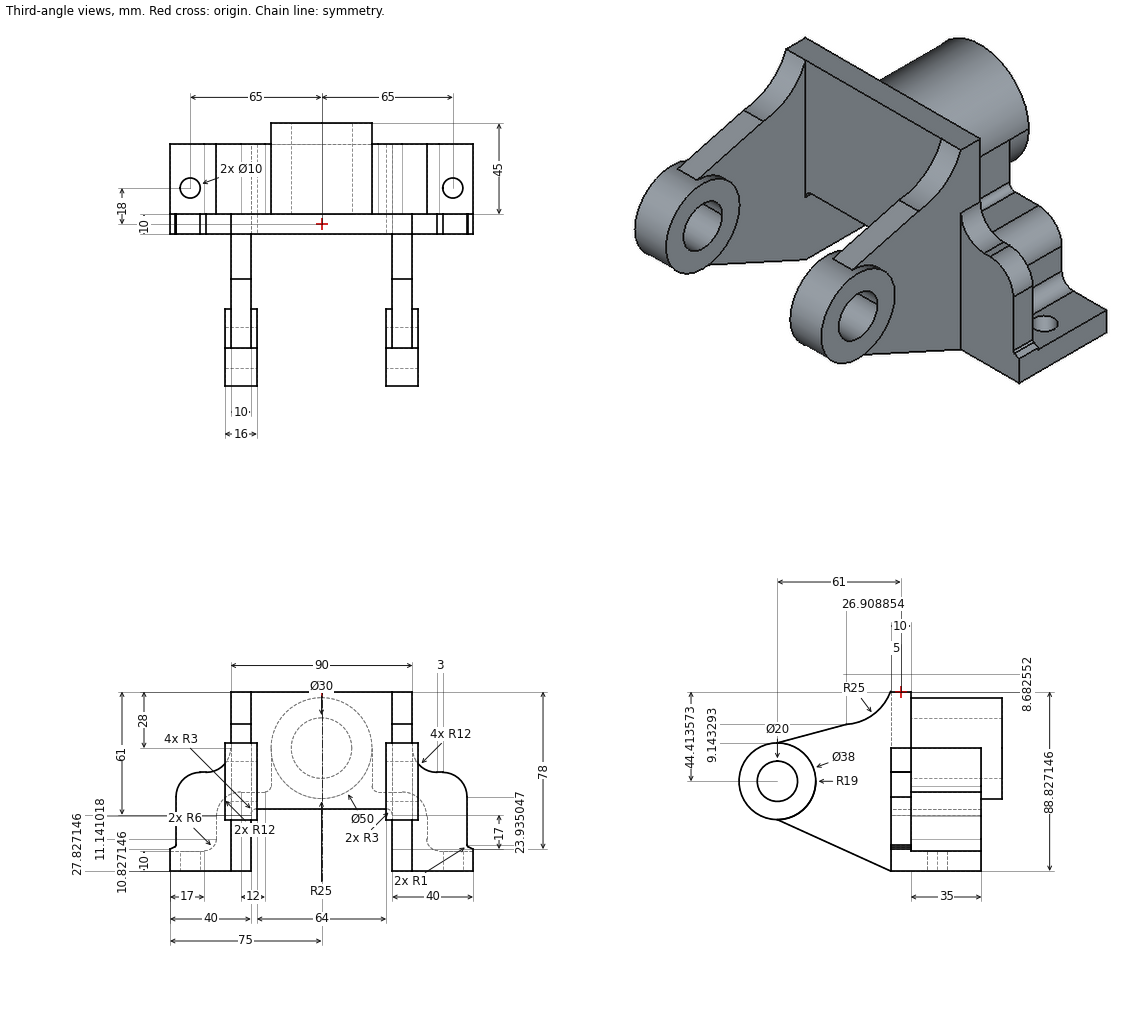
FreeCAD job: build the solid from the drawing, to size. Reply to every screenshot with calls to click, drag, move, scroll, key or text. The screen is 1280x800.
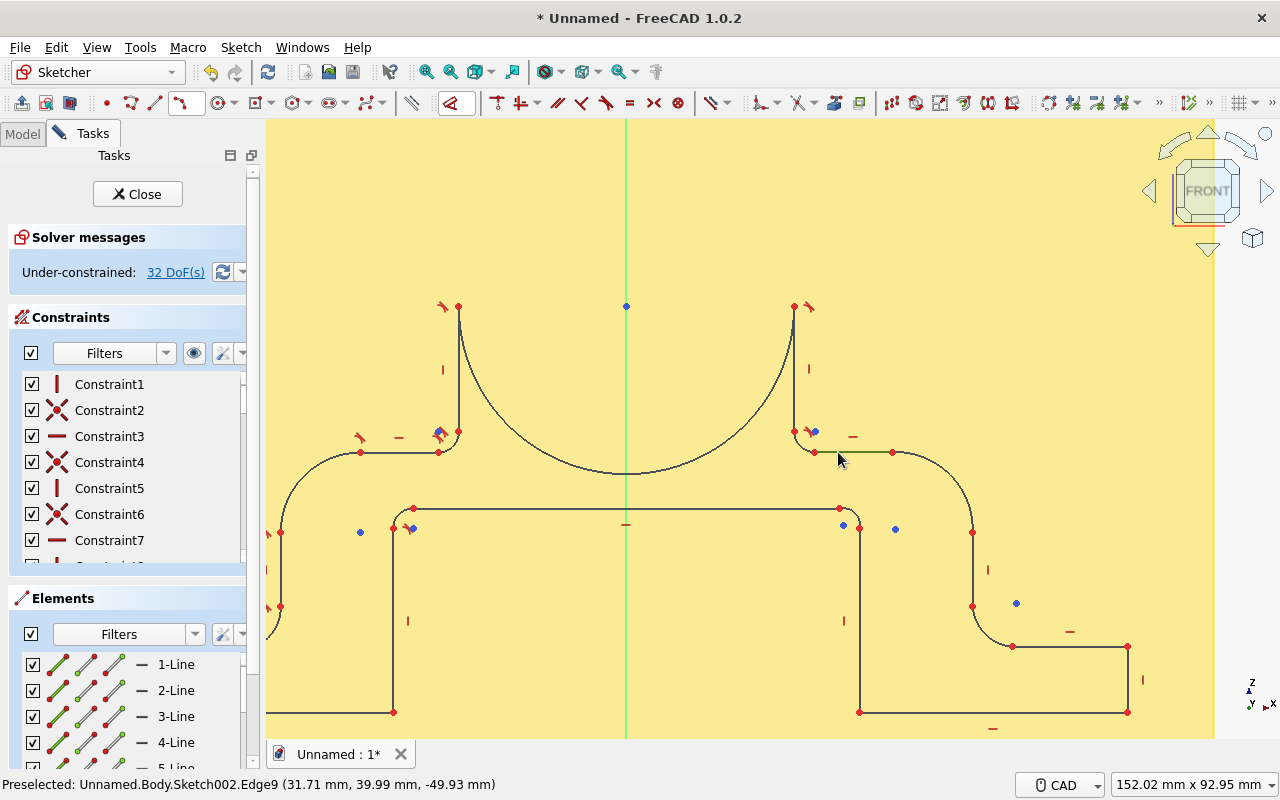
scroll(796, 440, up, 2)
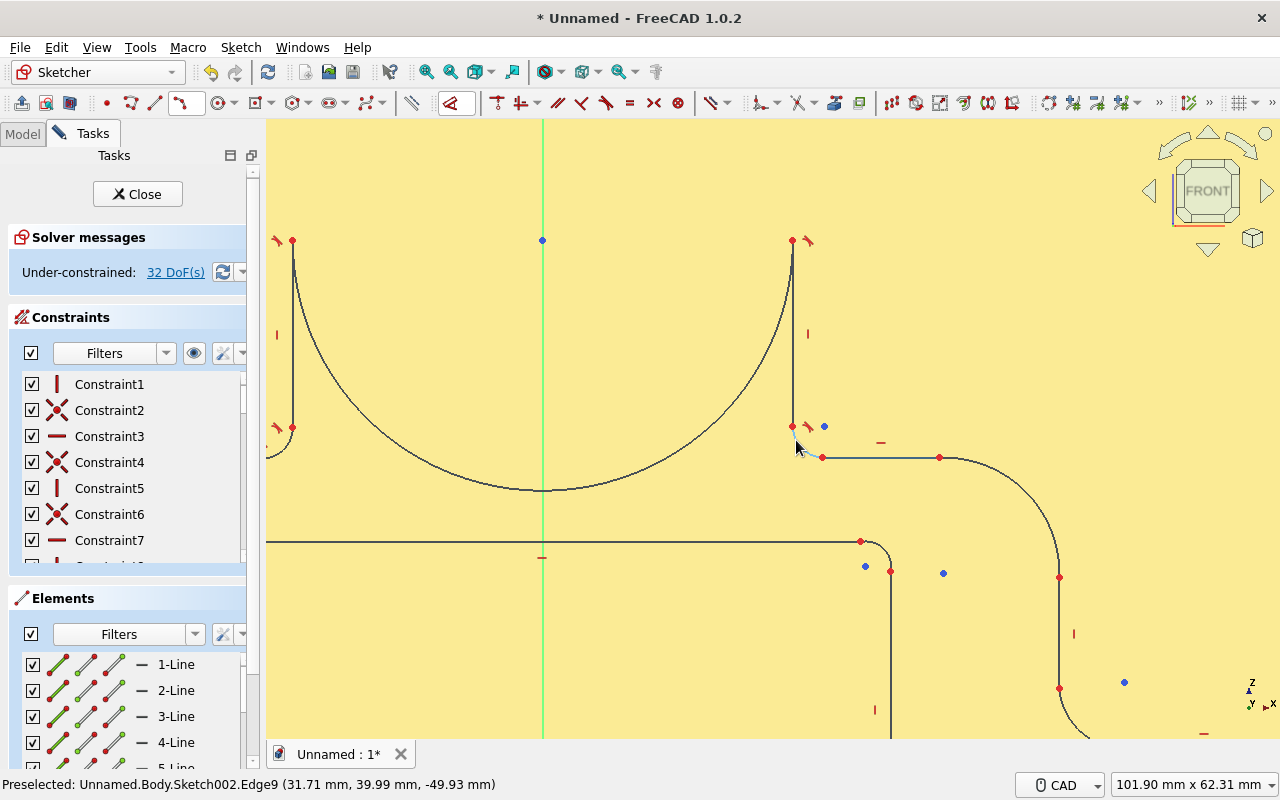
click(796, 440)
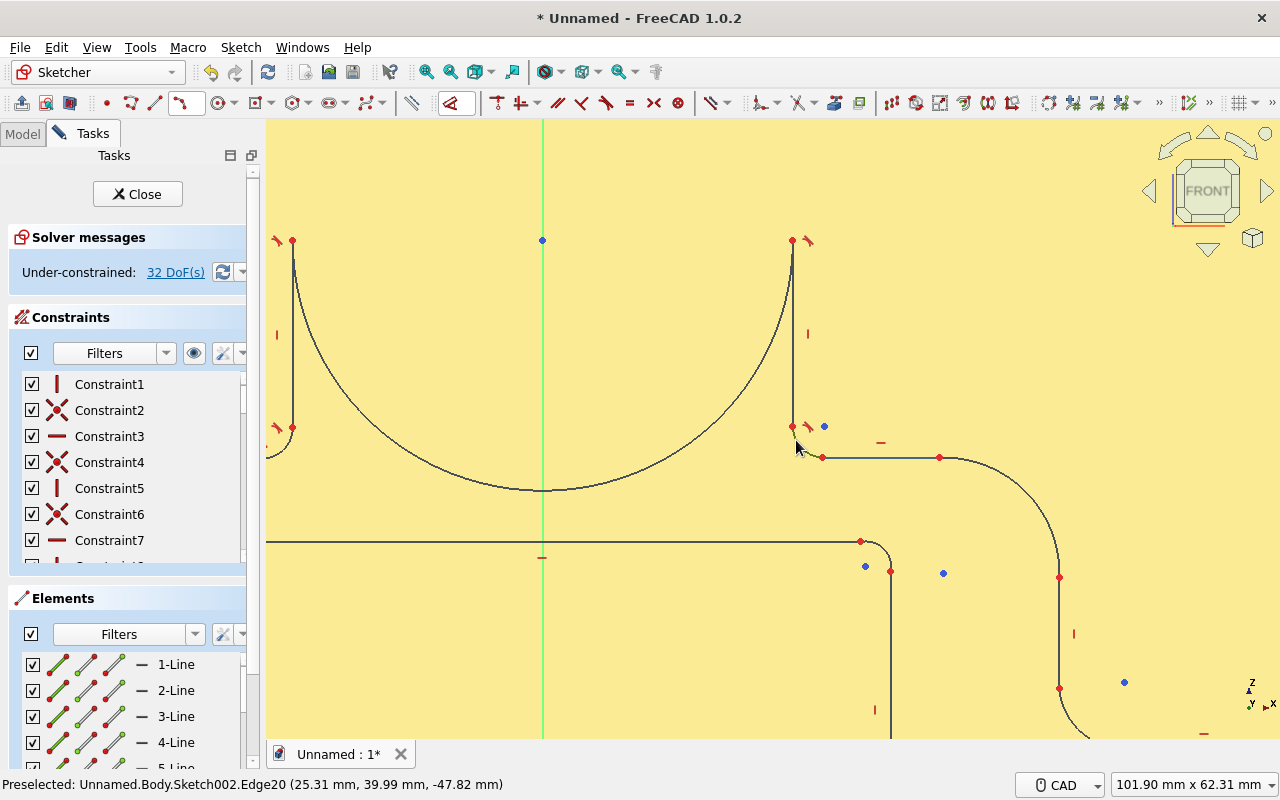
key(t)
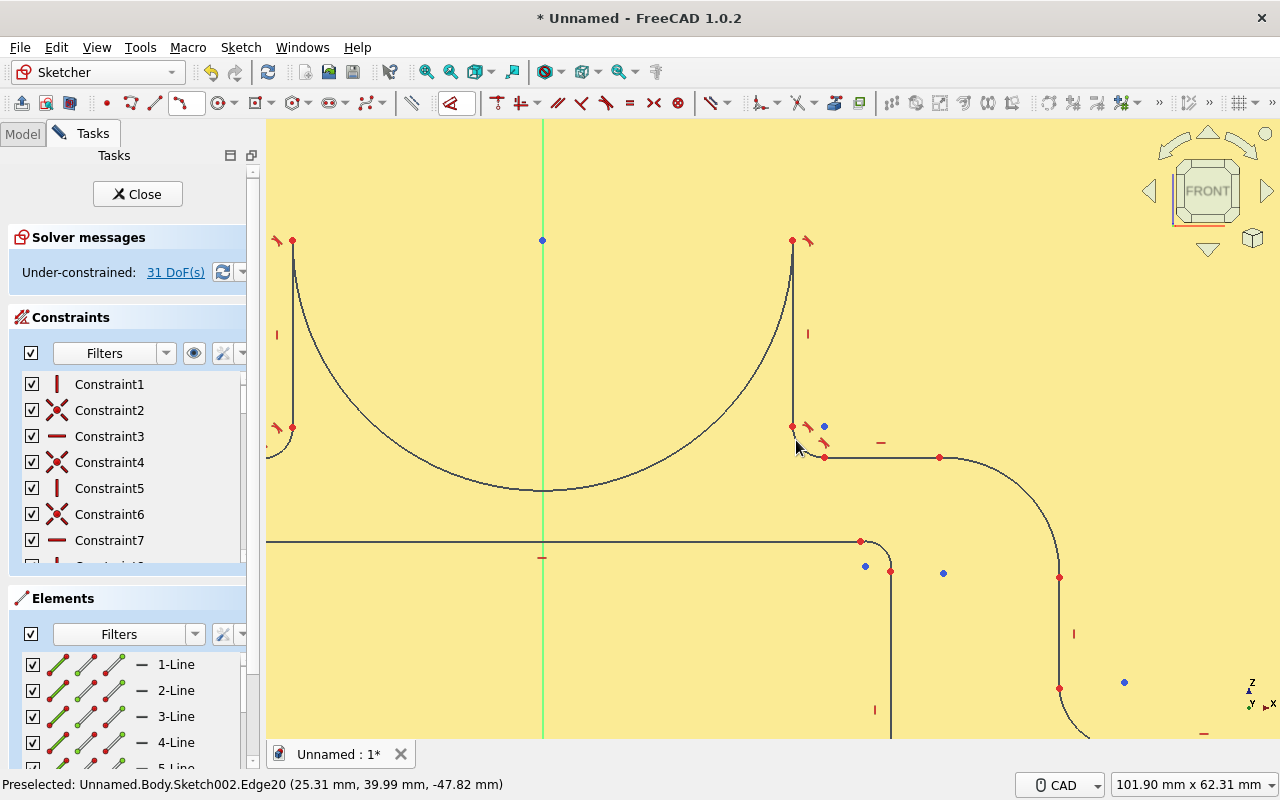
click(859, 458)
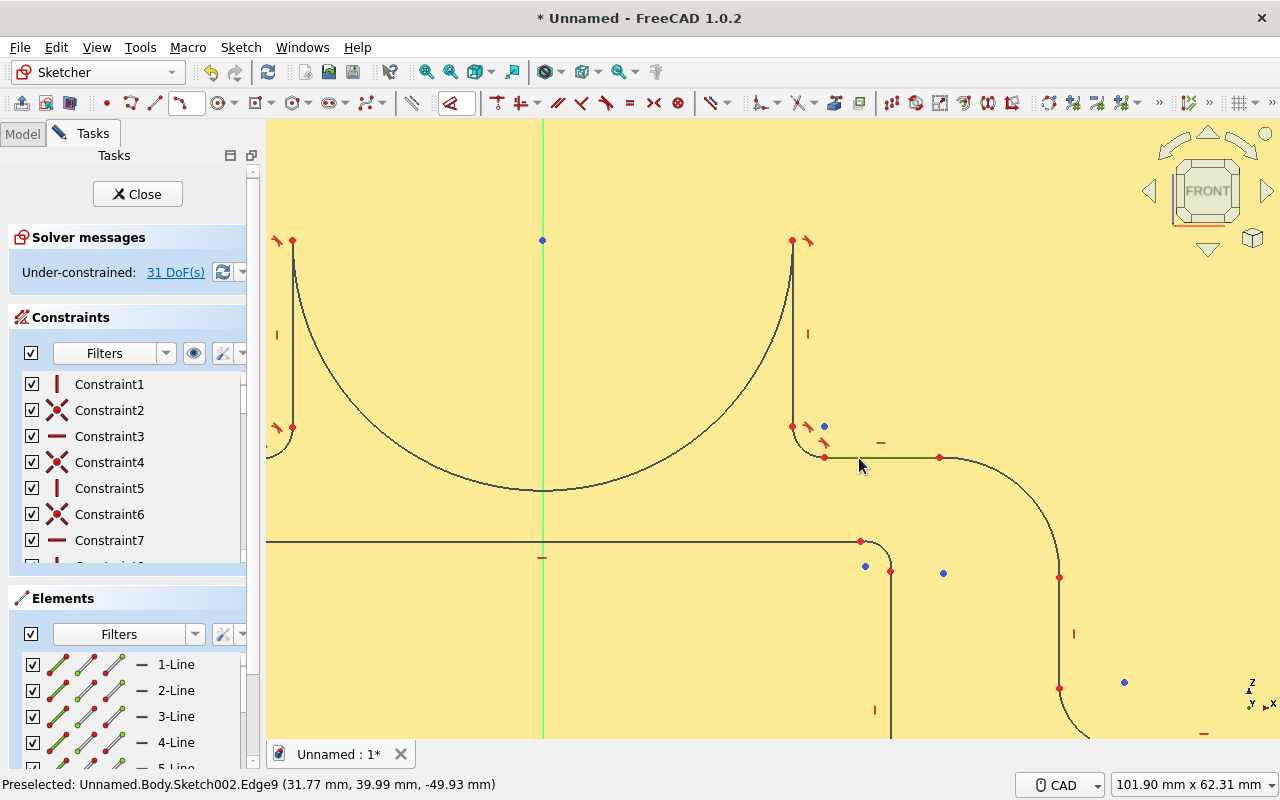
click(1047, 522)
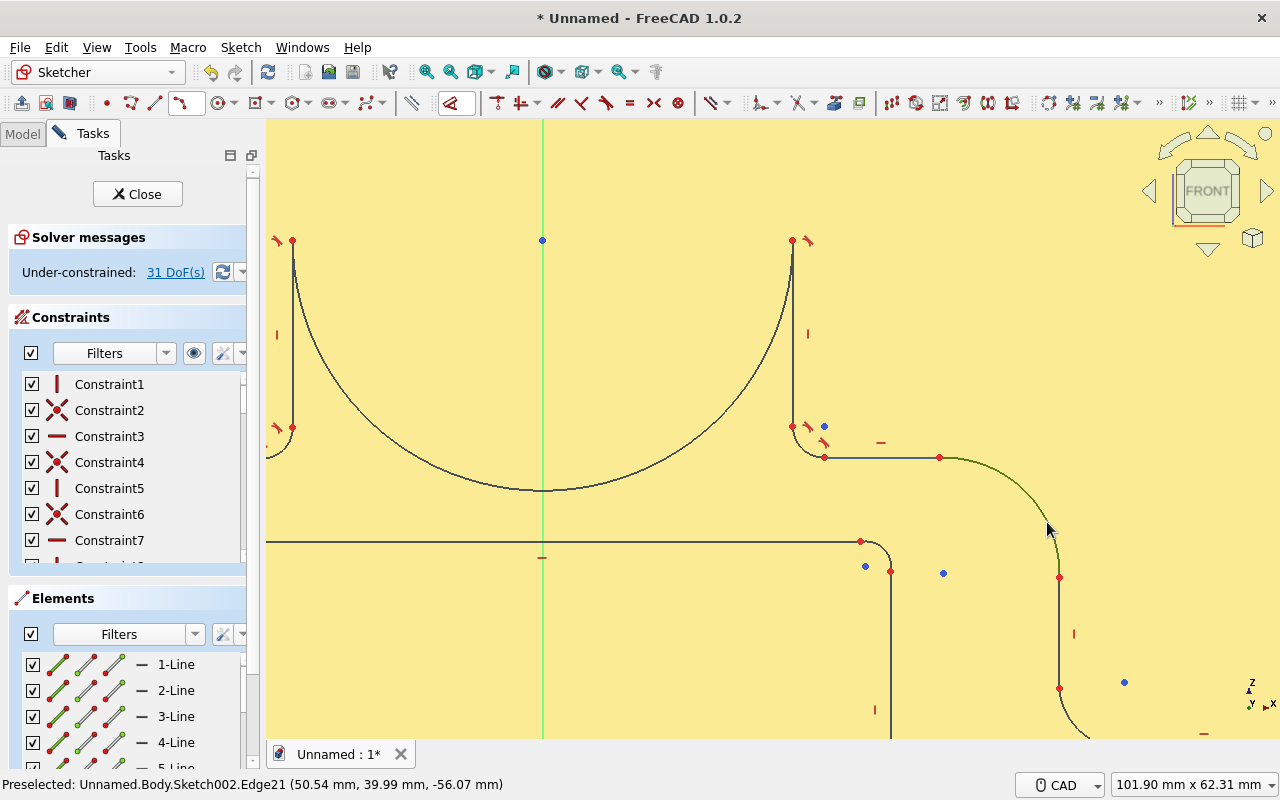
key(t)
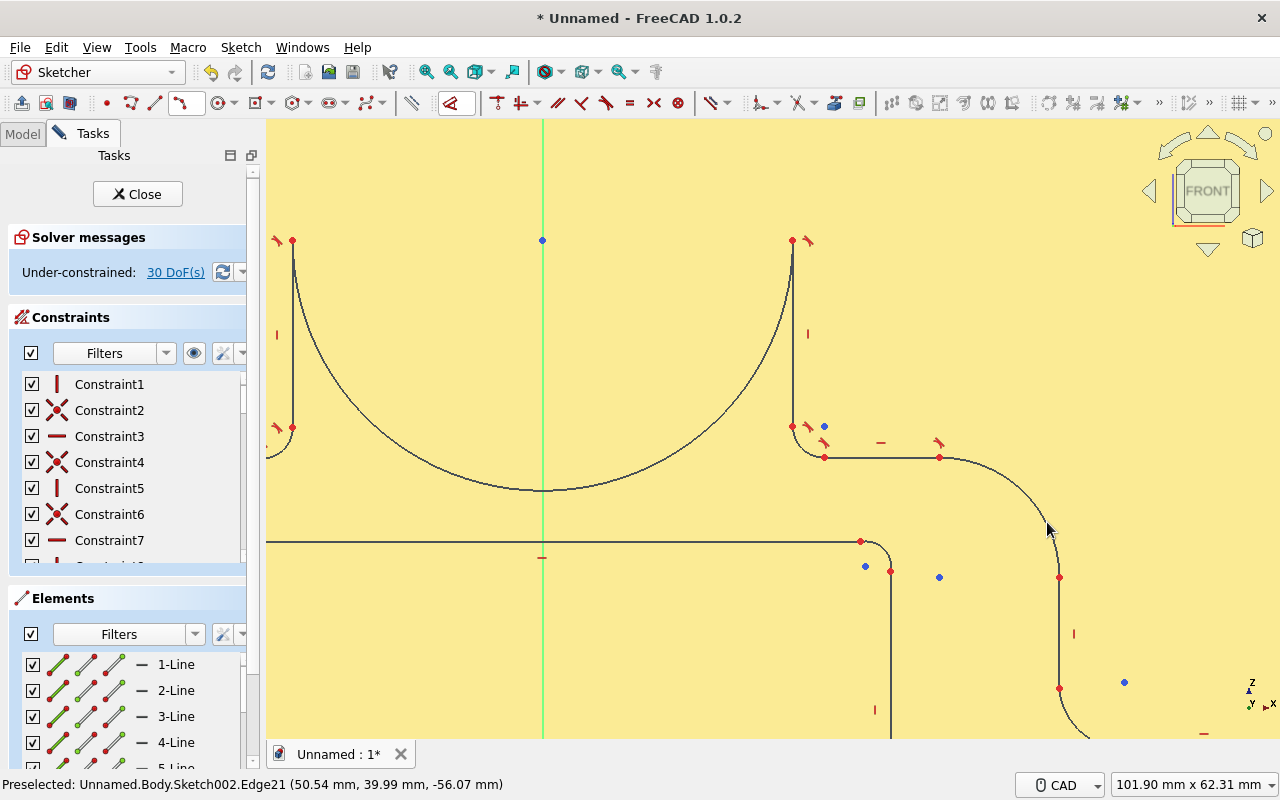
click(1059, 611)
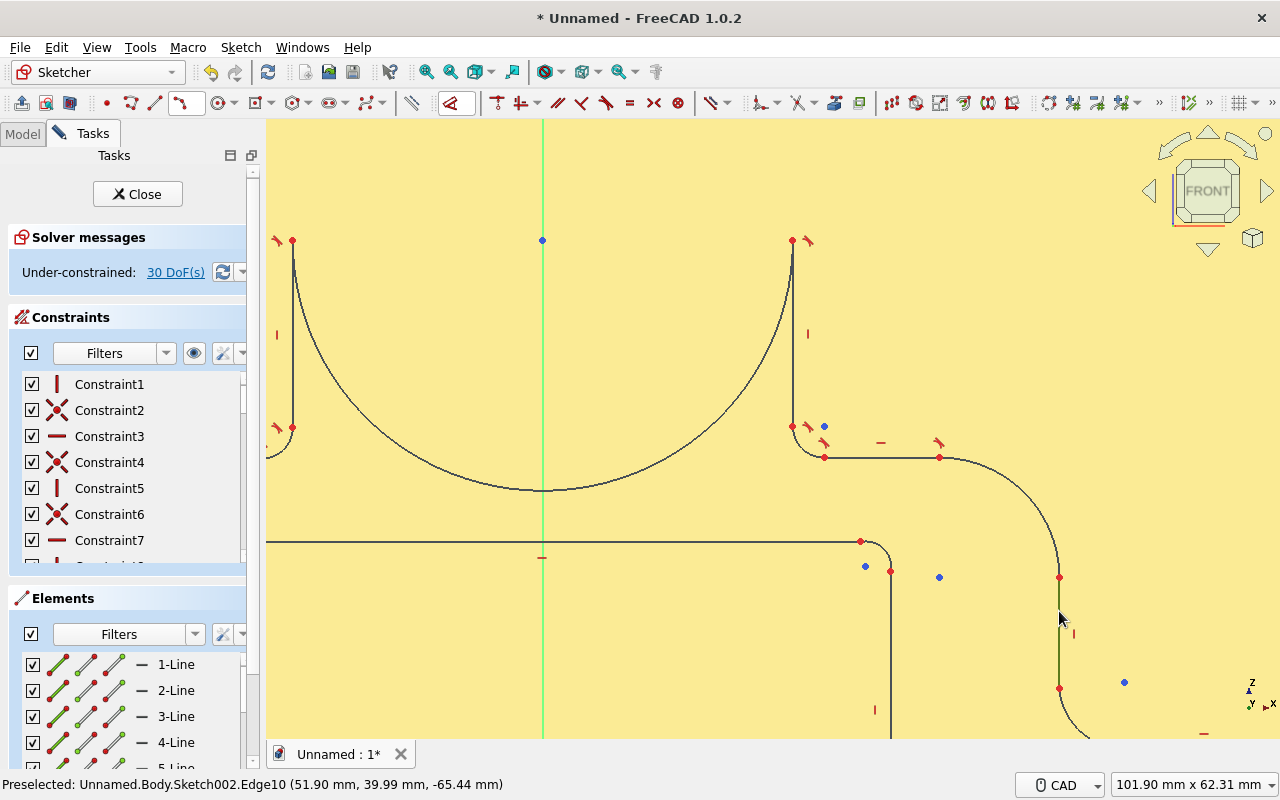
click(1046, 523)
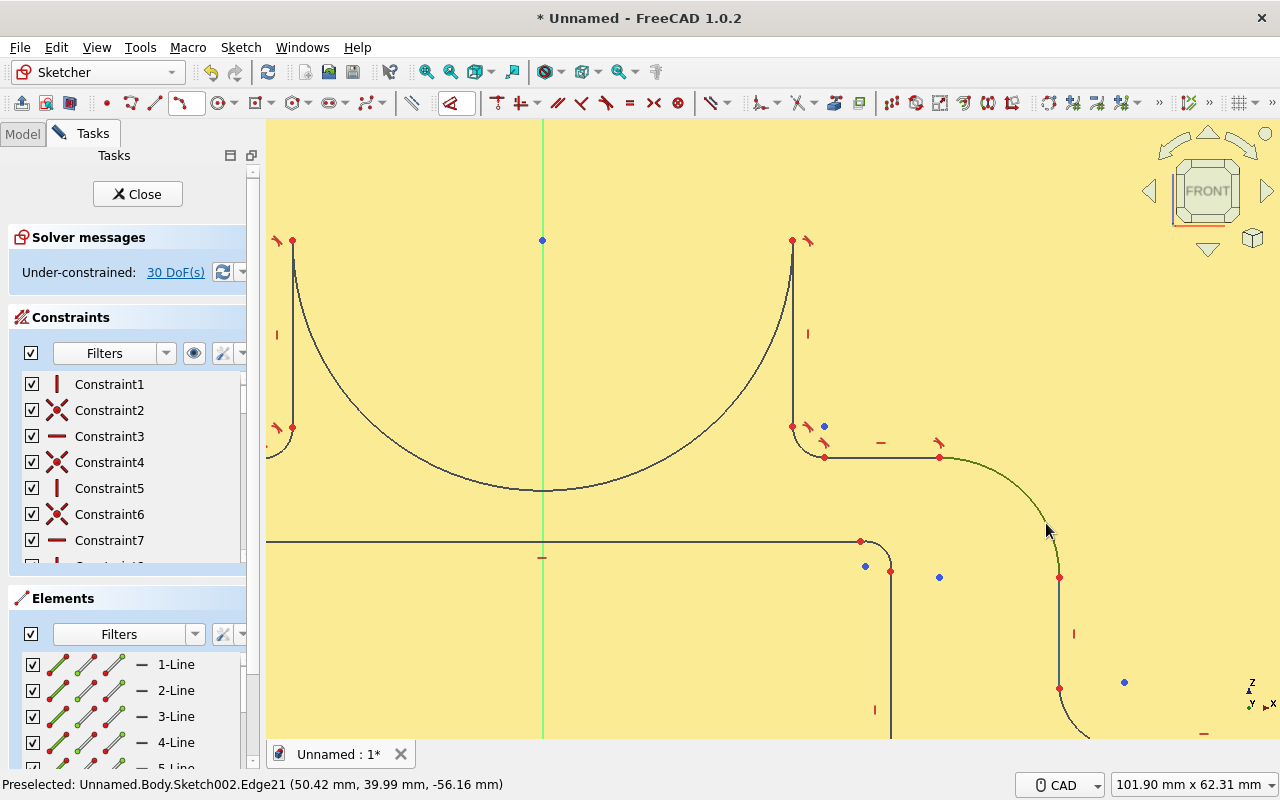
click(606, 104)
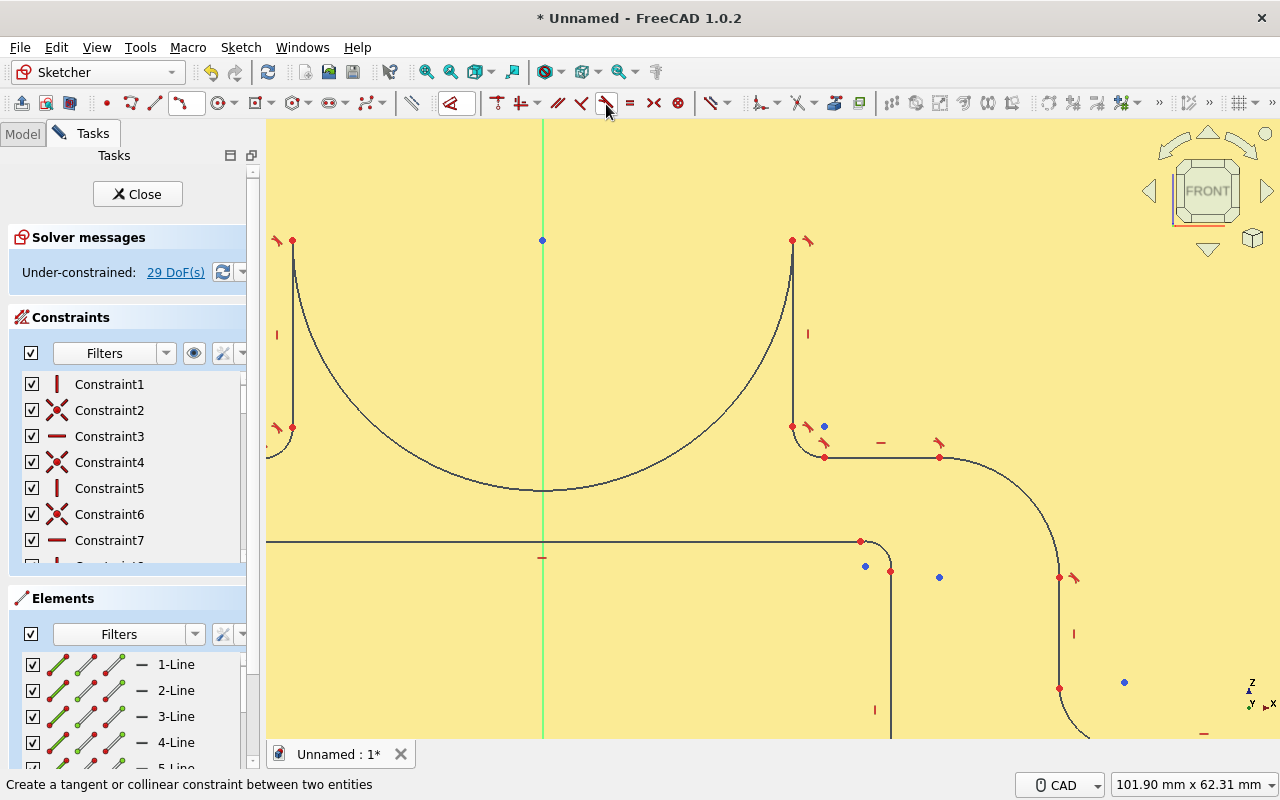
click(1059, 611)